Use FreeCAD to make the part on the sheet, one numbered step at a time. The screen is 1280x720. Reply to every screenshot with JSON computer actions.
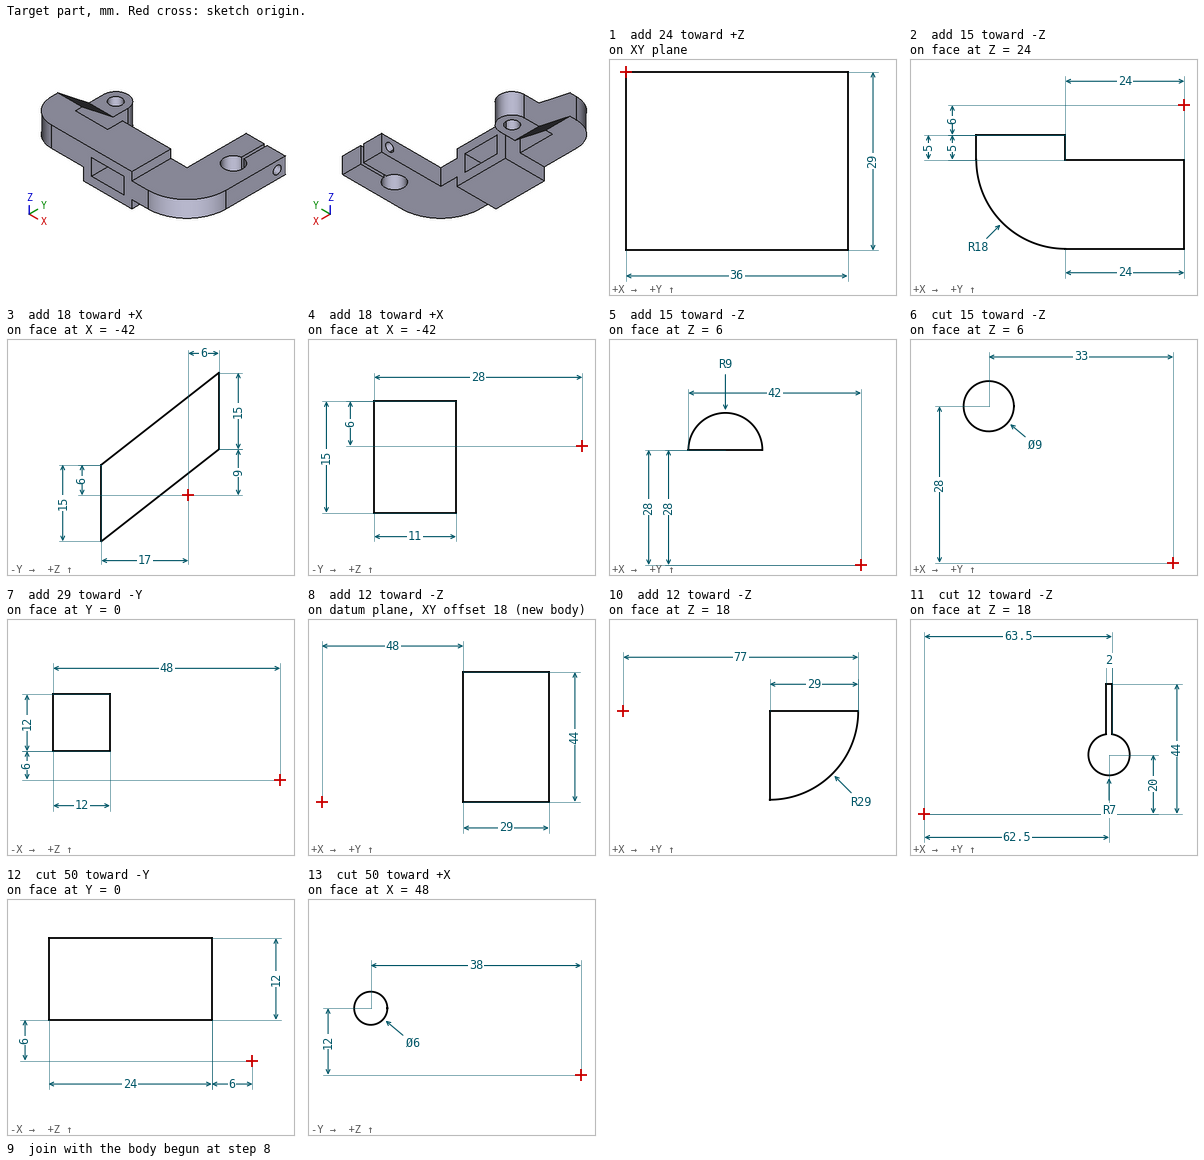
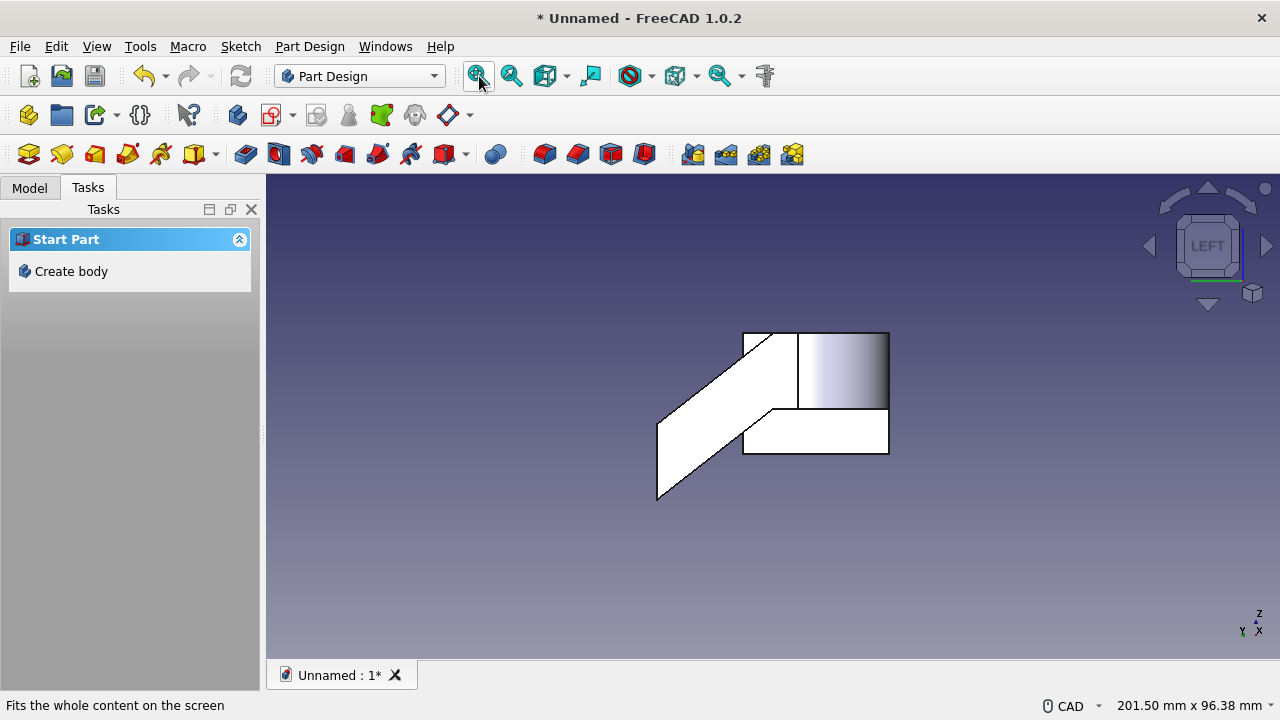
{"action": "left_click", "coordinate": [748, 392]}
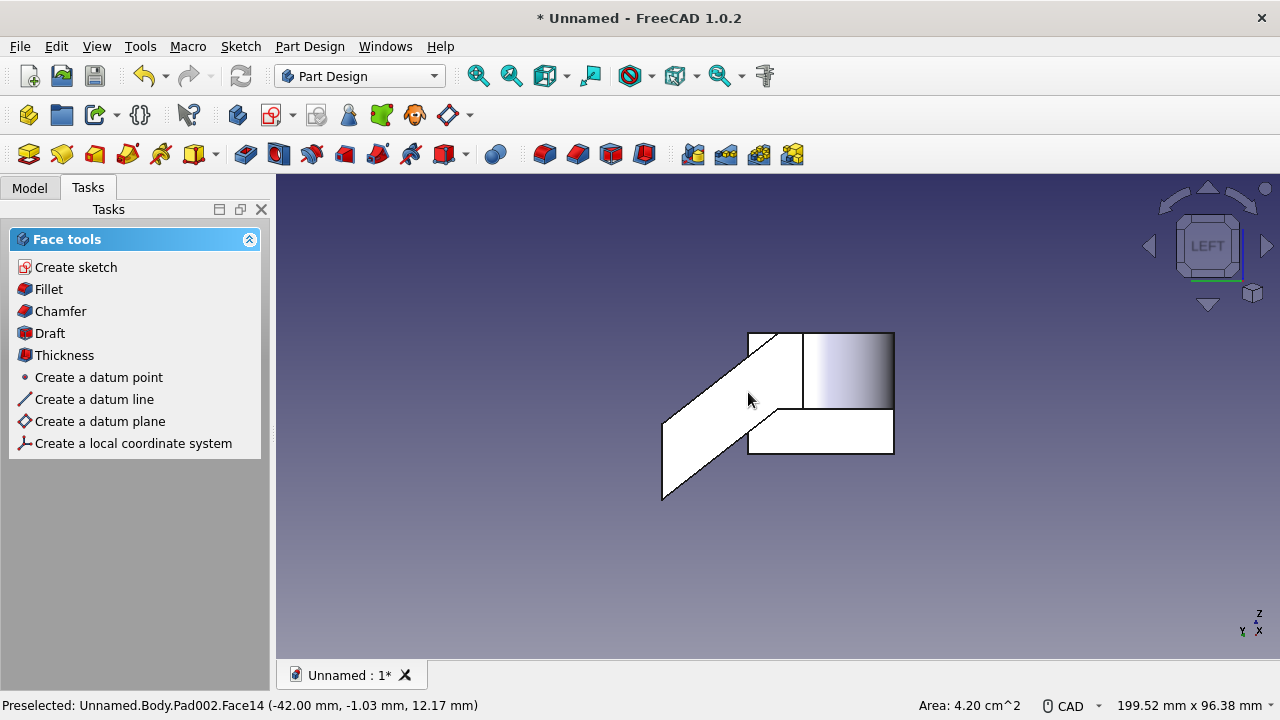
{"action": "left_click", "coordinate": [270, 116]}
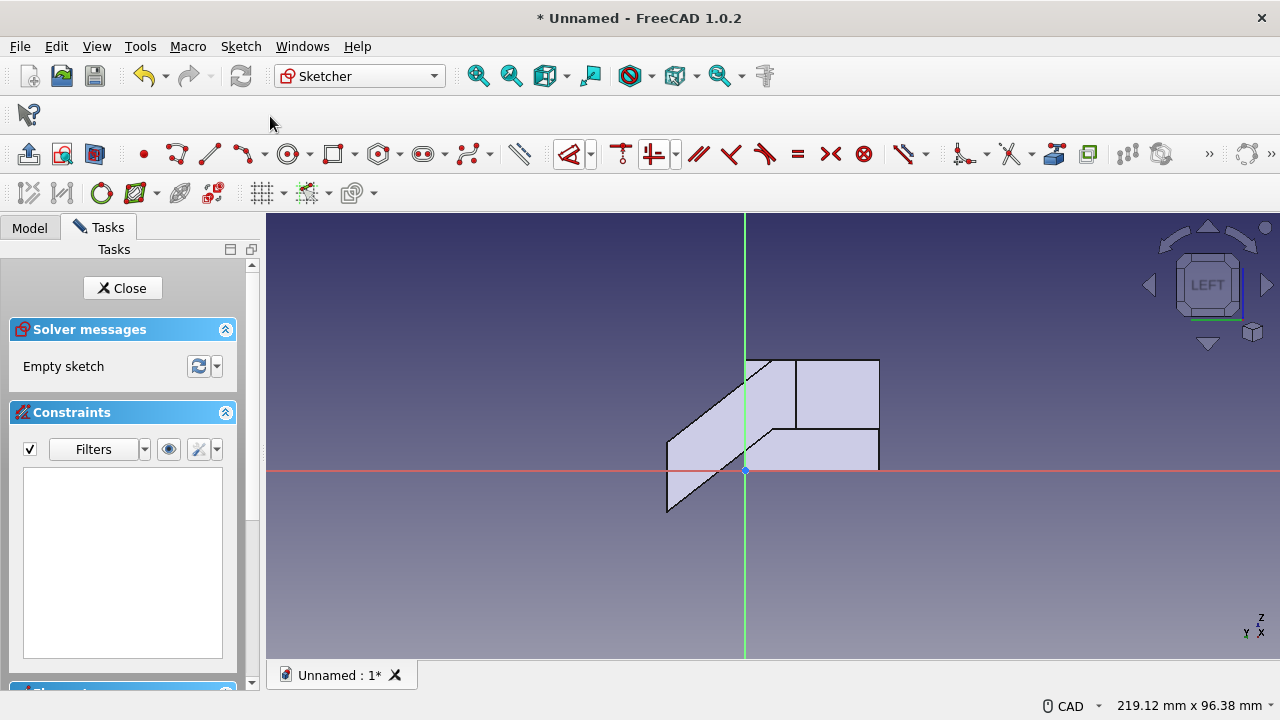
{"action": "scroll", "coordinate": [673, 491], "scroll_direction": "up", "scroll_amount": 7}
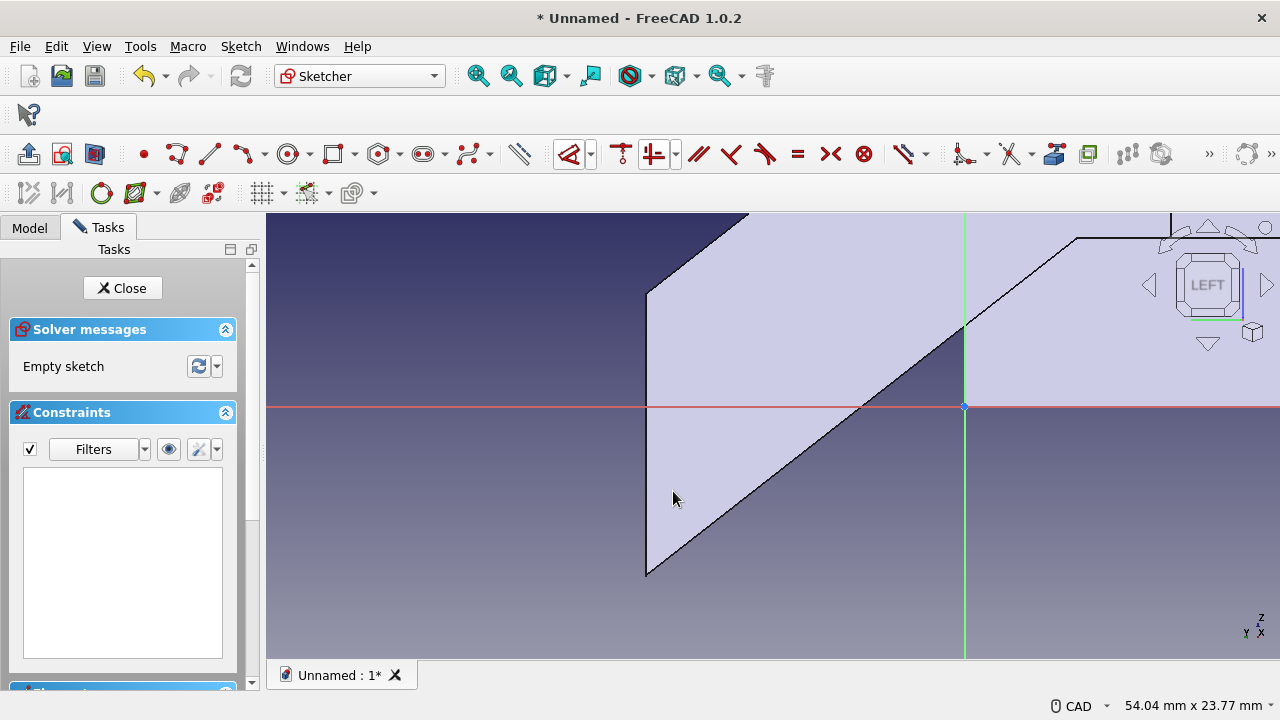
{"action": "left_click", "coordinate": [332, 154]}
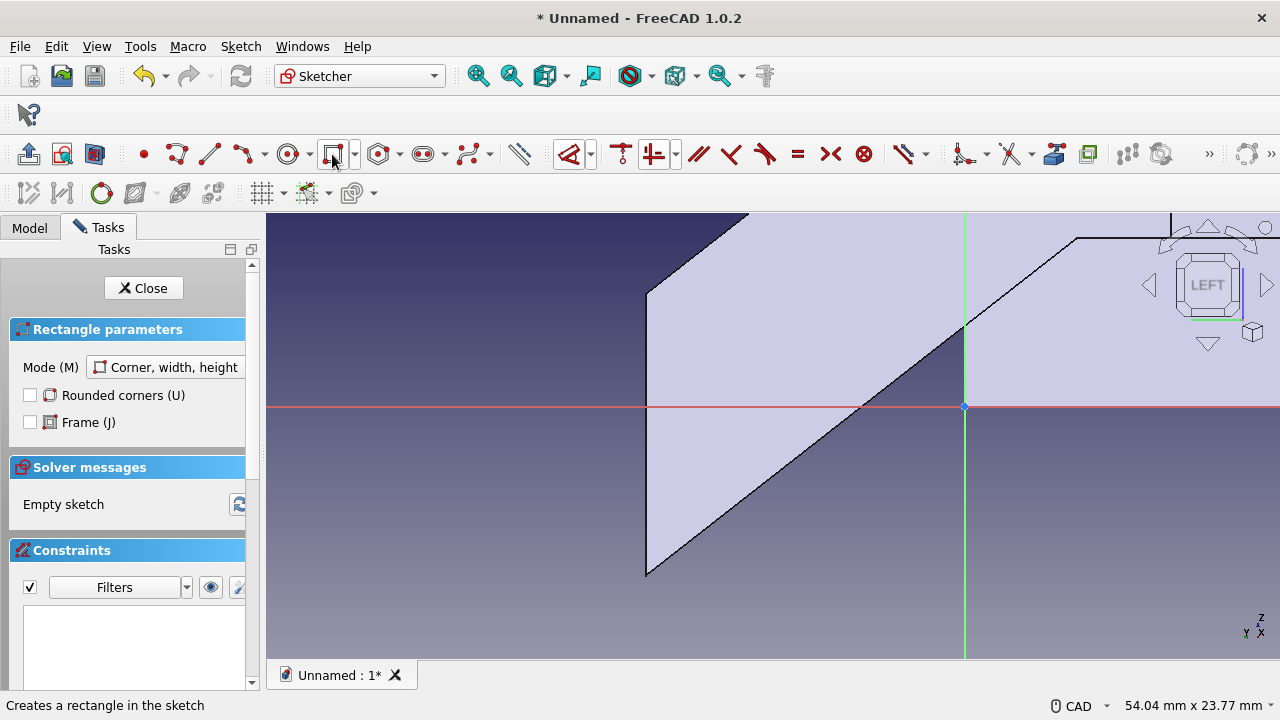
{"action": "left_click", "coordinate": [439, 294]}
{"action": "mouse_move", "coordinate": [646, 576]}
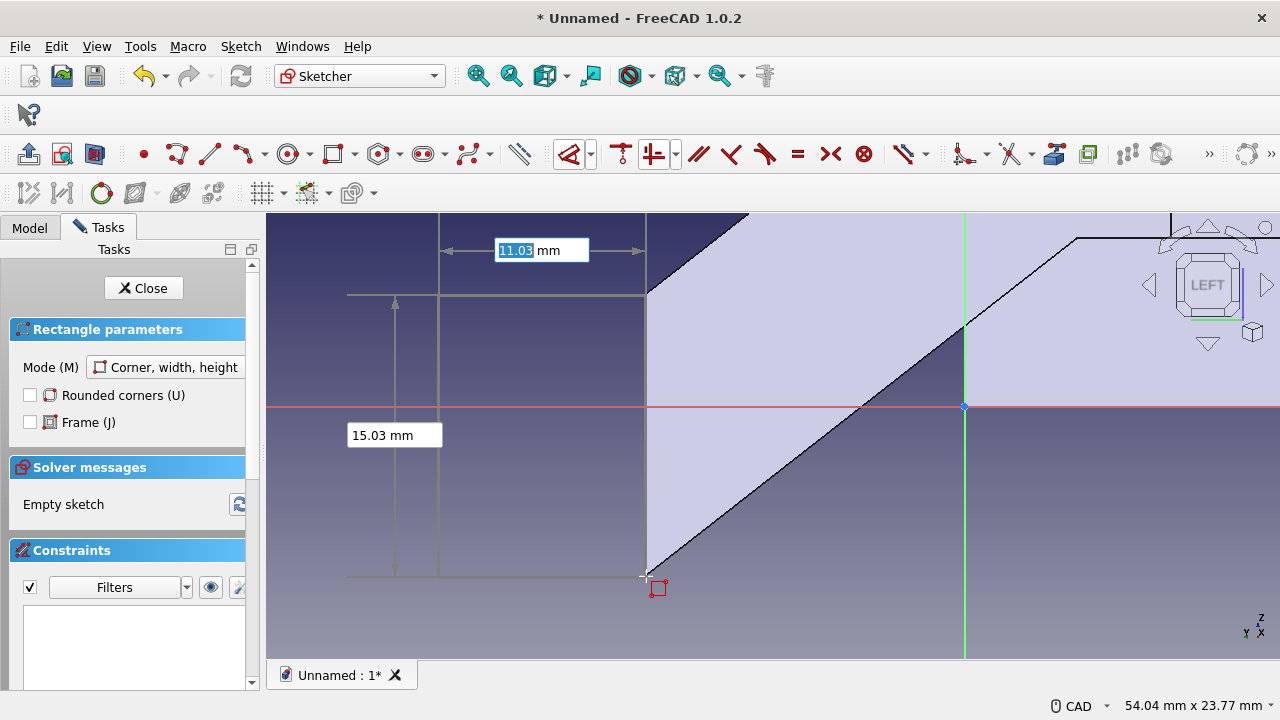
{"action": "type", "text": "11"}
{"action": "key", "text": "Tab"}
{"action": "type", "text": "15"}
{"action": "key", "text": "Return"}
{"action": "key", "text": "Escape"}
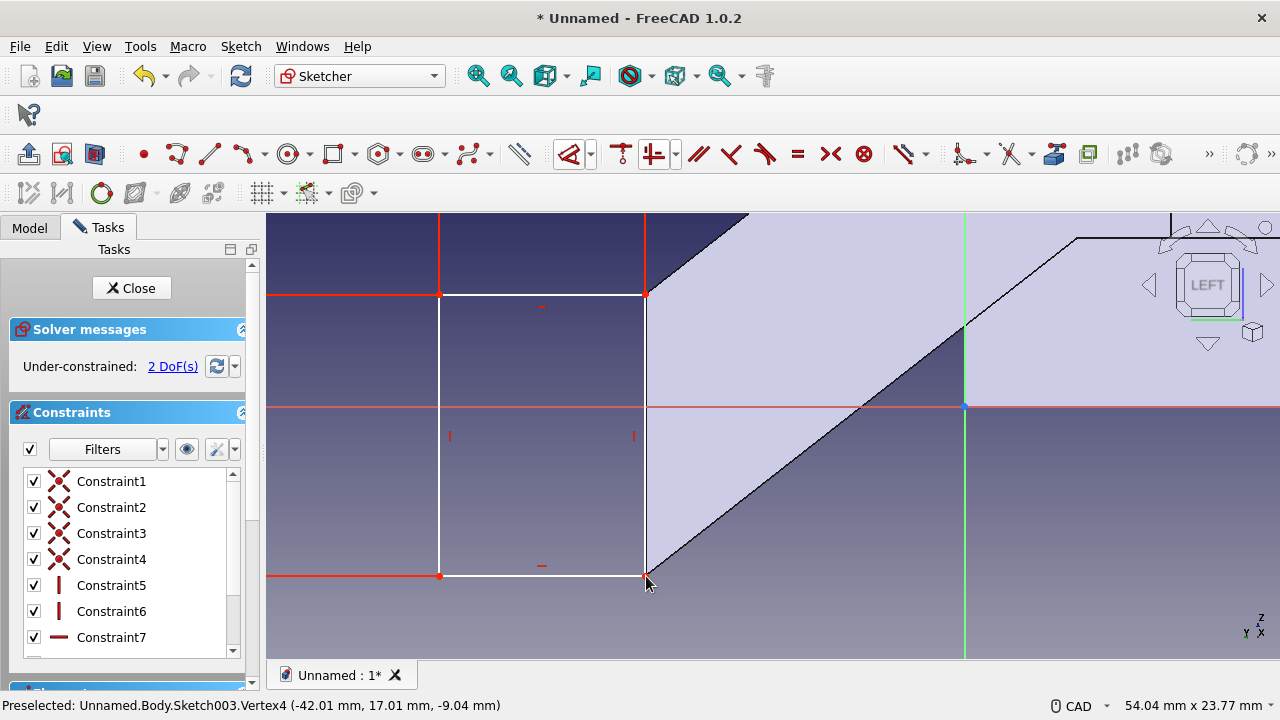
{"action": "left_click", "coordinate": [439, 295]}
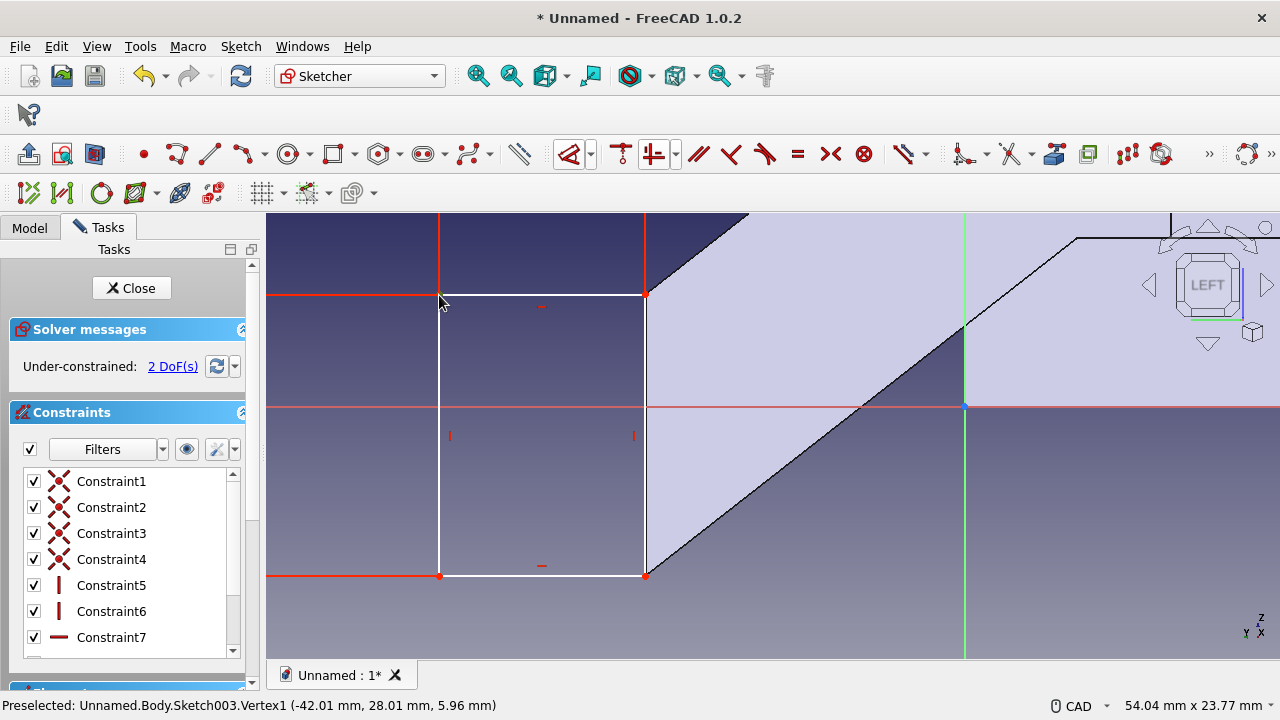
{"action": "left_click", "coordinate": [590, 154]}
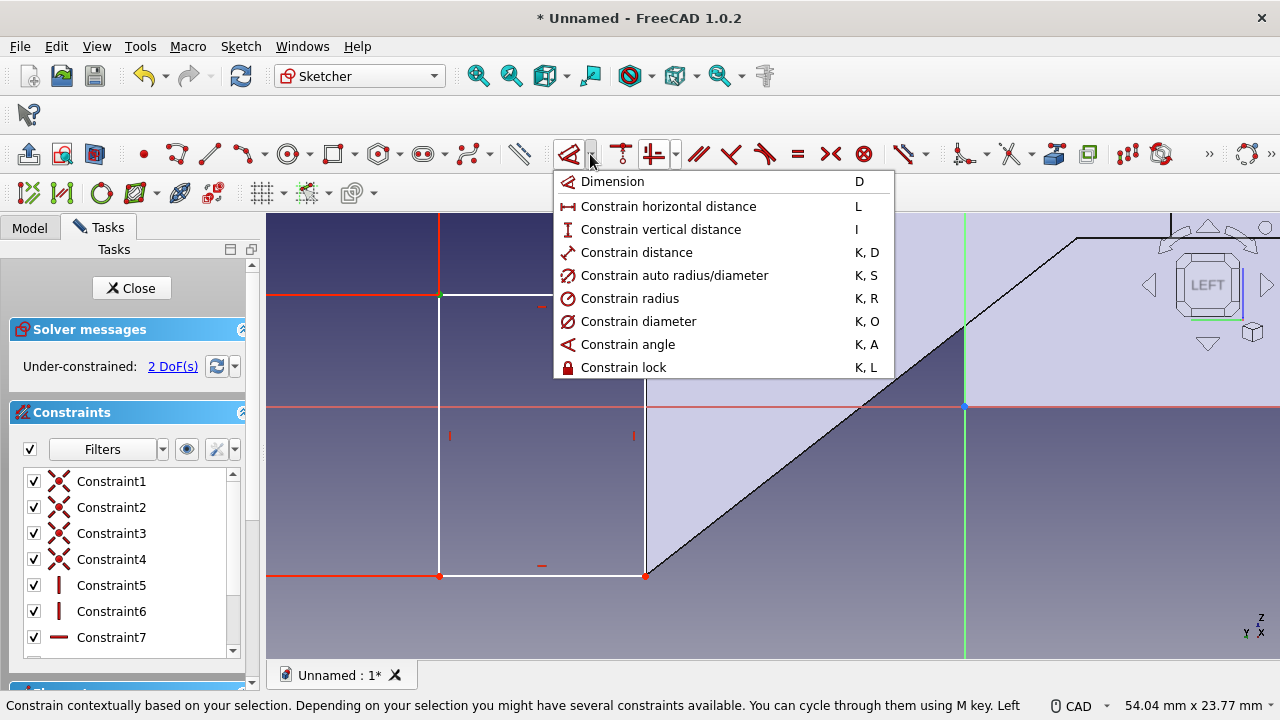
{"action": "left_click", "coordinate": [724, 230]}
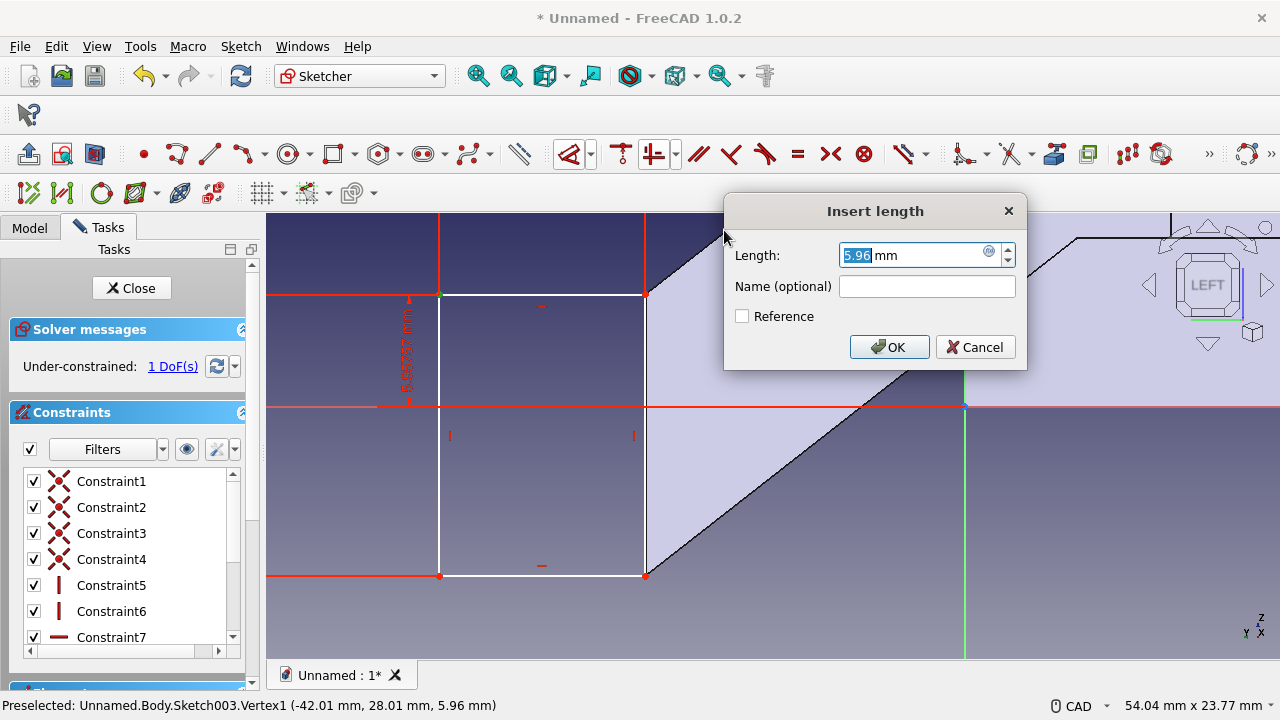
{"action": "type", "text": "6"}
{"action": "key", "text": "Return"}